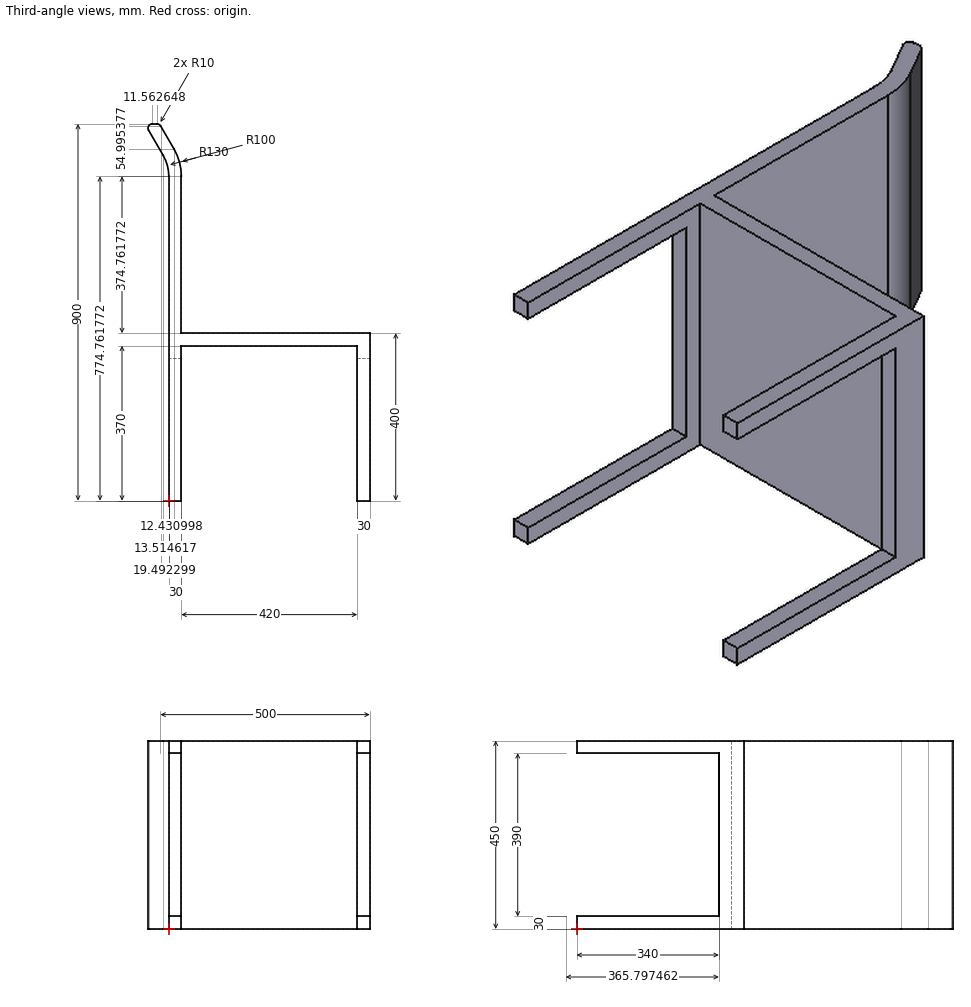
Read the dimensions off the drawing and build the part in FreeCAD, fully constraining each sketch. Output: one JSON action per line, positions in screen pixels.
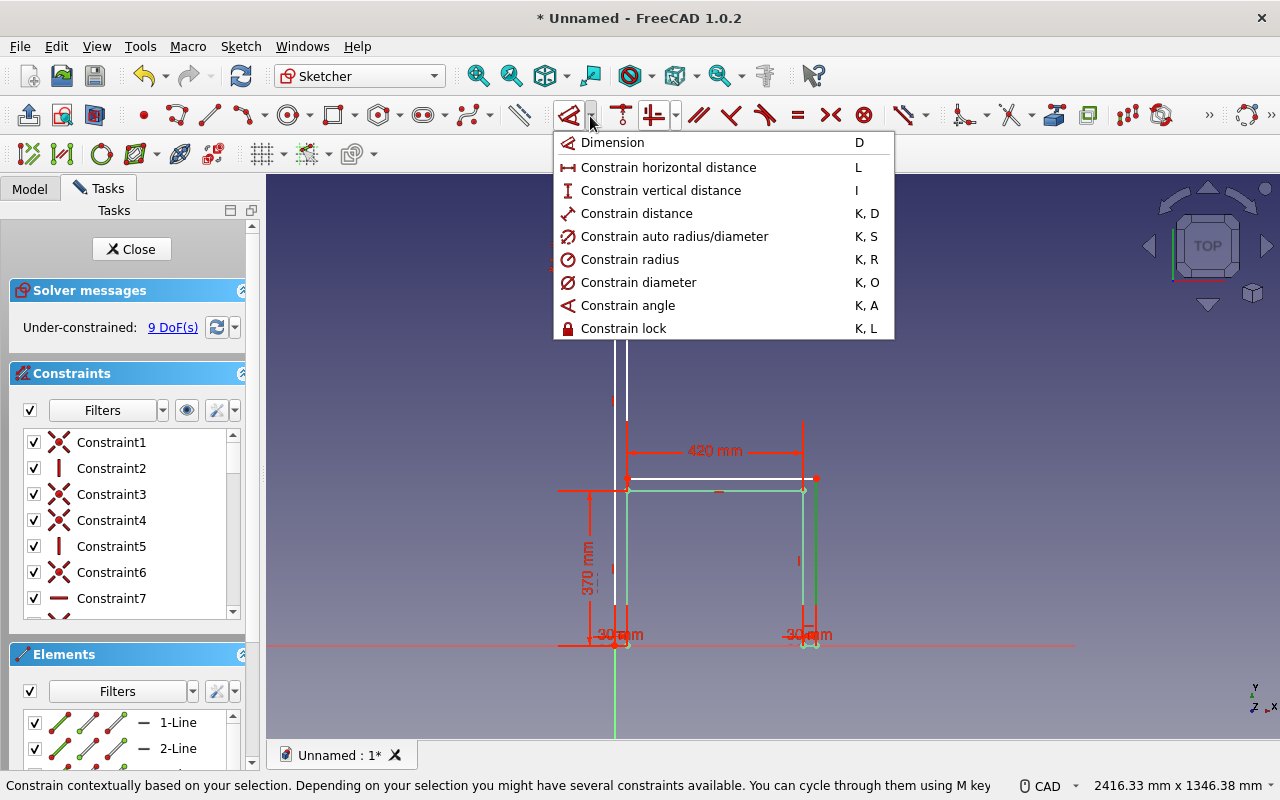
{"action": "left_click", "coordinate": [724, 190]}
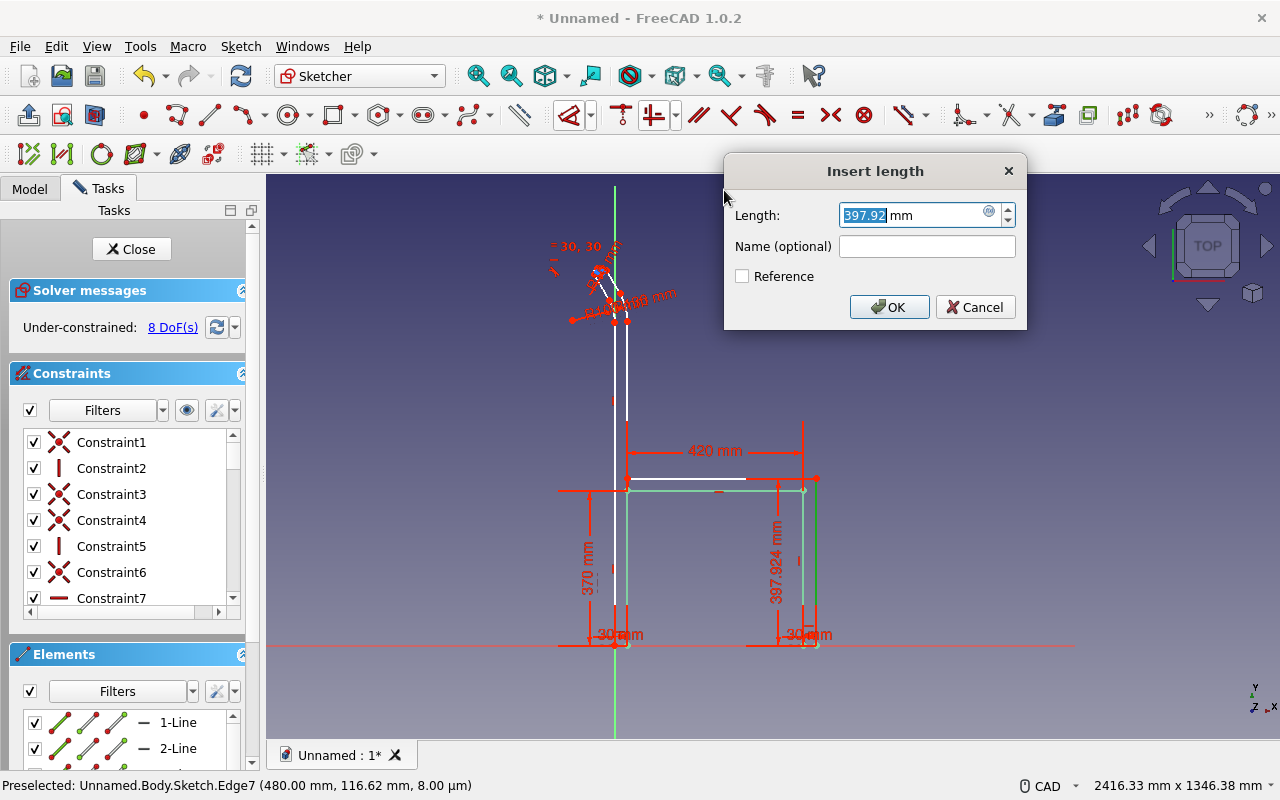
{"action": "type", "text": "400"}
{"action": "key", "text": "Return"}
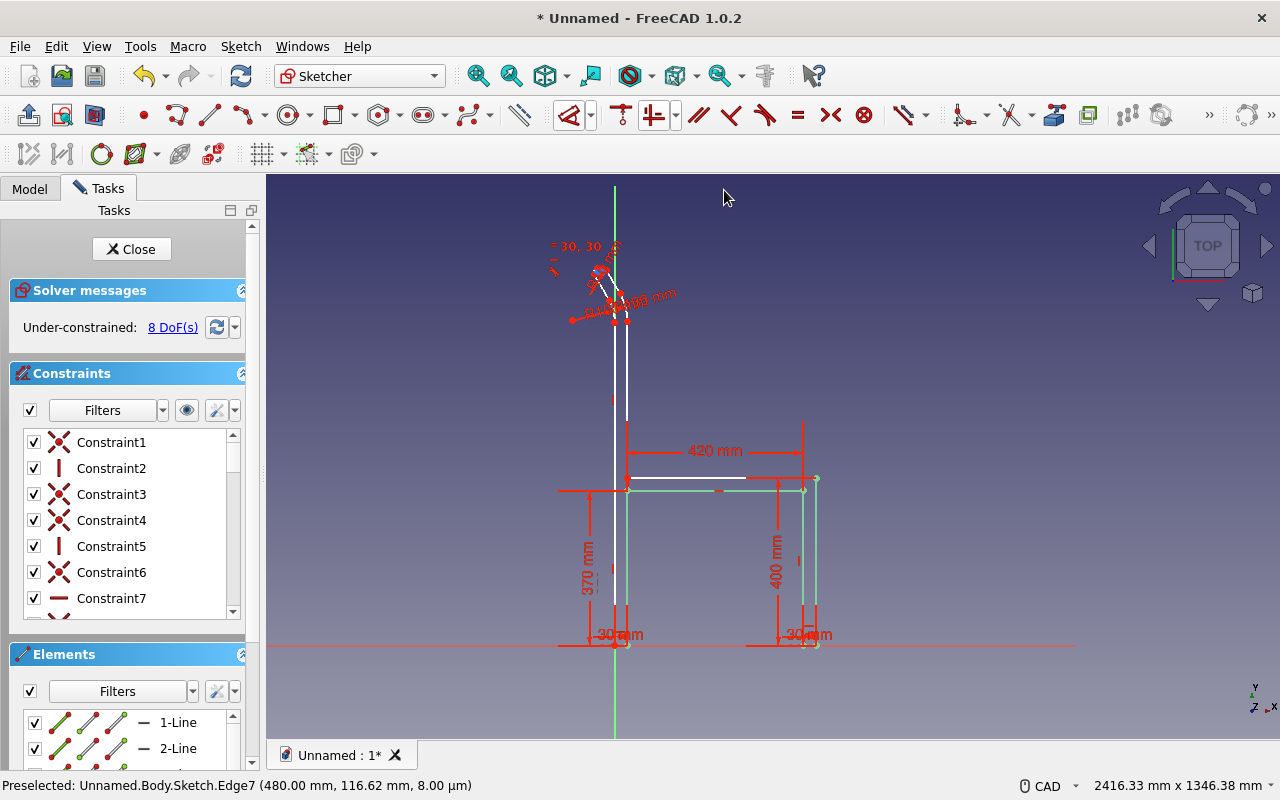
{"action": "scroll", "coordinate": [603, 269], "scroll_direction": "up", "scroll_amount": 6}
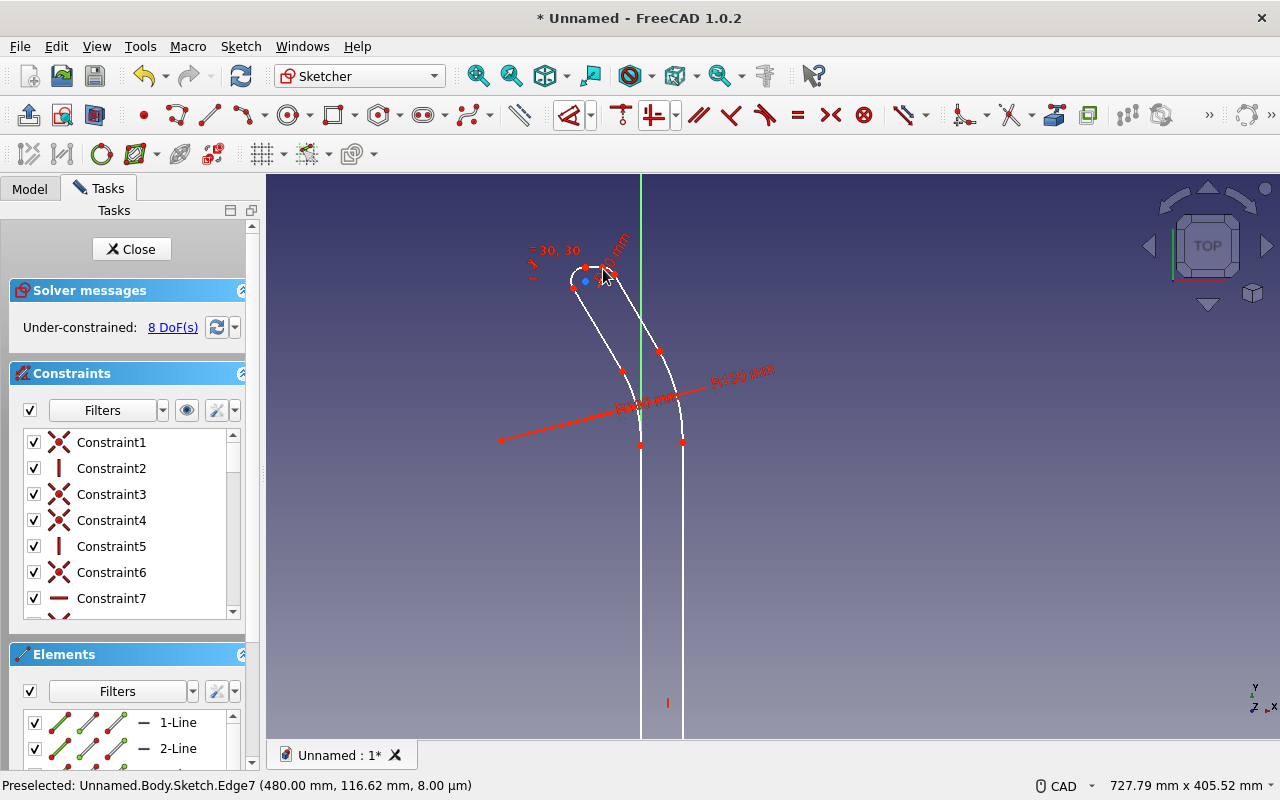
{"action": "left_click", "coordinate": [602, 267]}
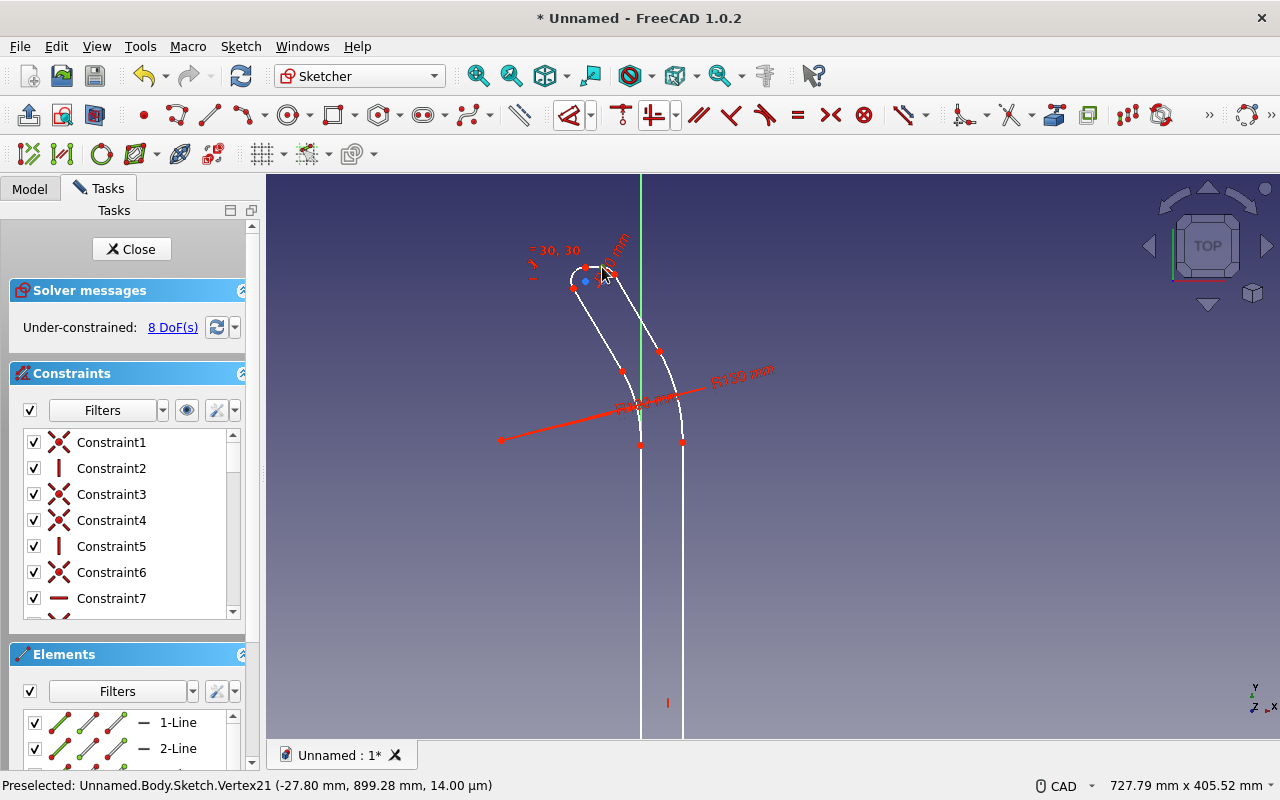
{"action": "key", "text": "i"}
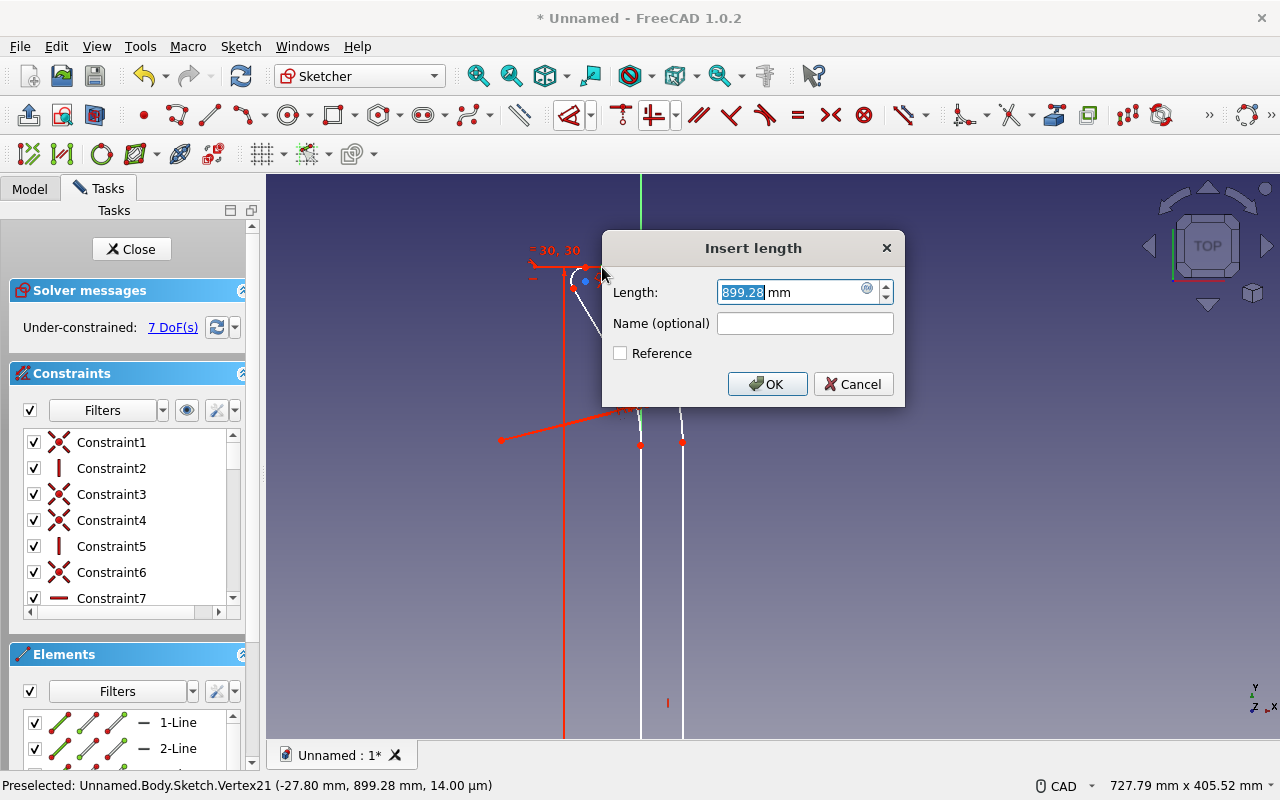
{"action": "type", "text": "900"}
{"action": "key", "text": "Return"}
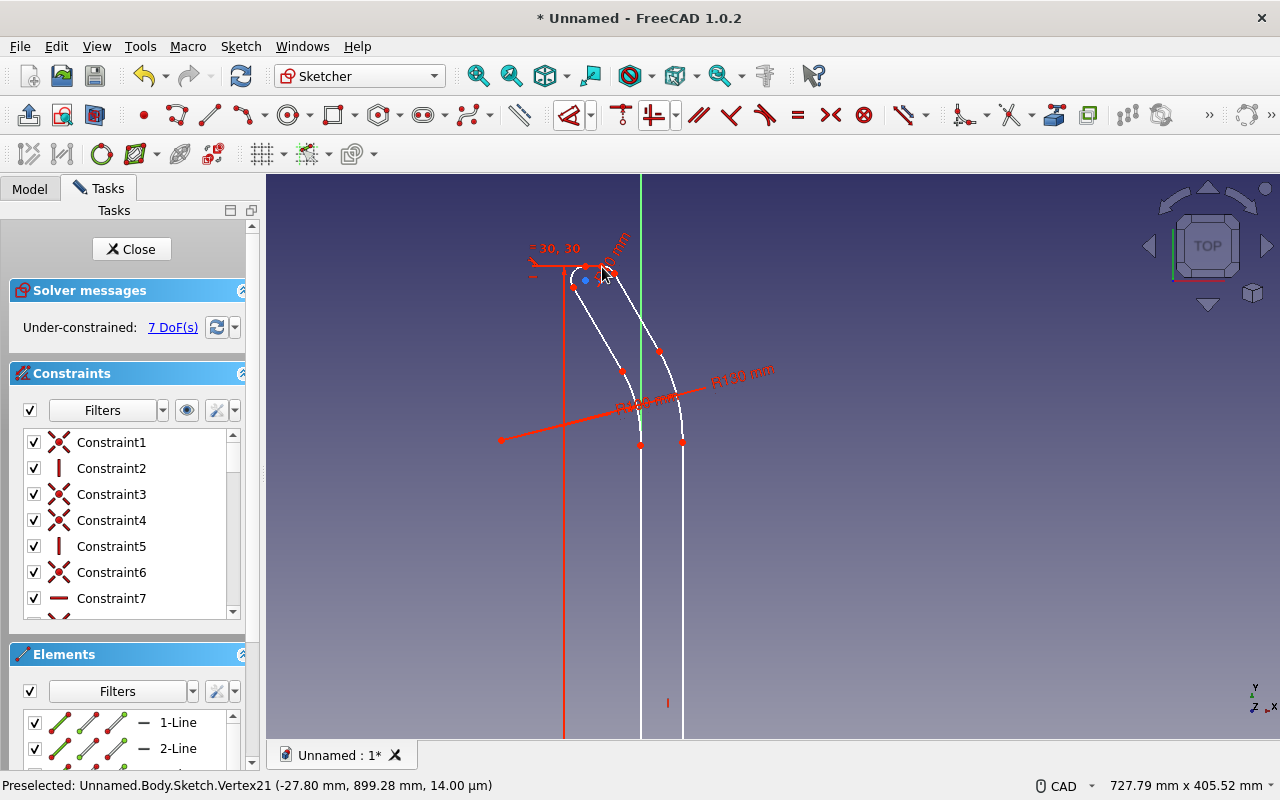
{"action": "scroll", "coordinate": [594, 266], "scroll_direction": "up", "scroll_amount": 5}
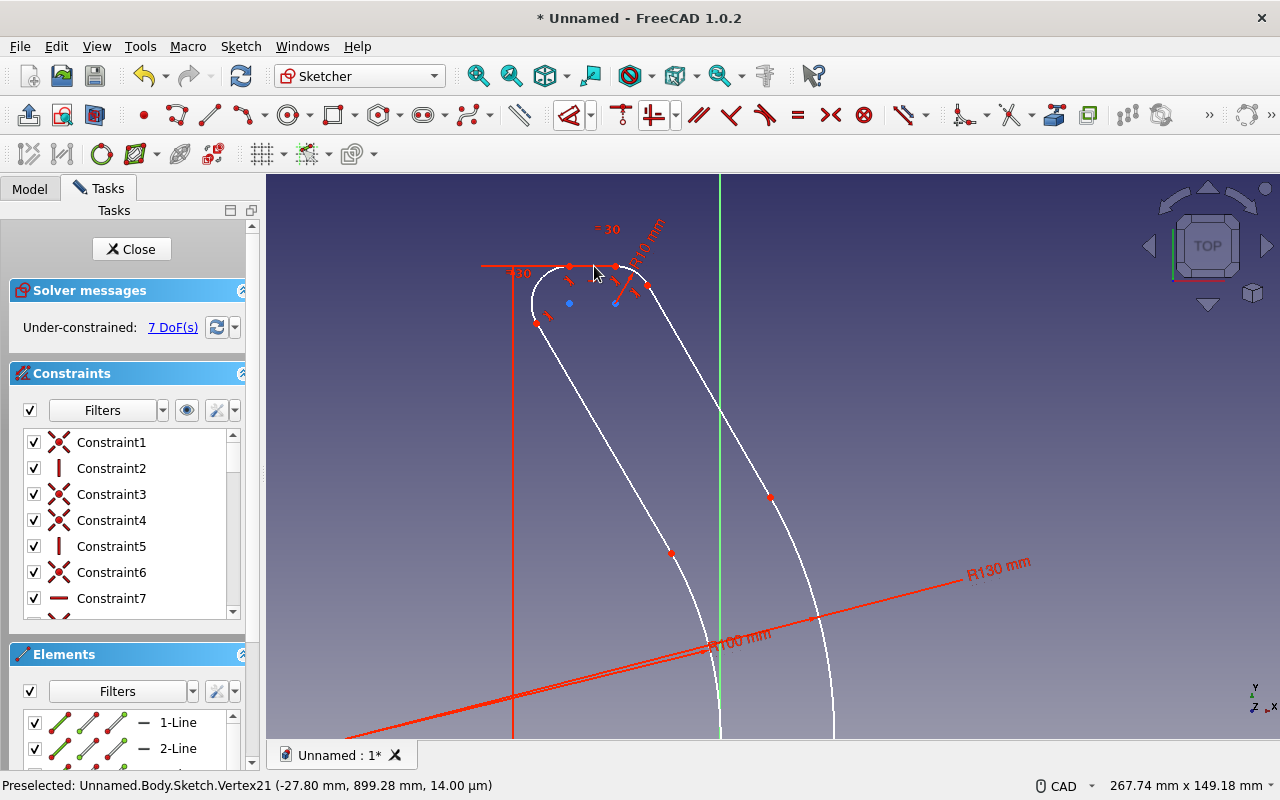
{"action": "left_click", "coordinate": [592, 266]}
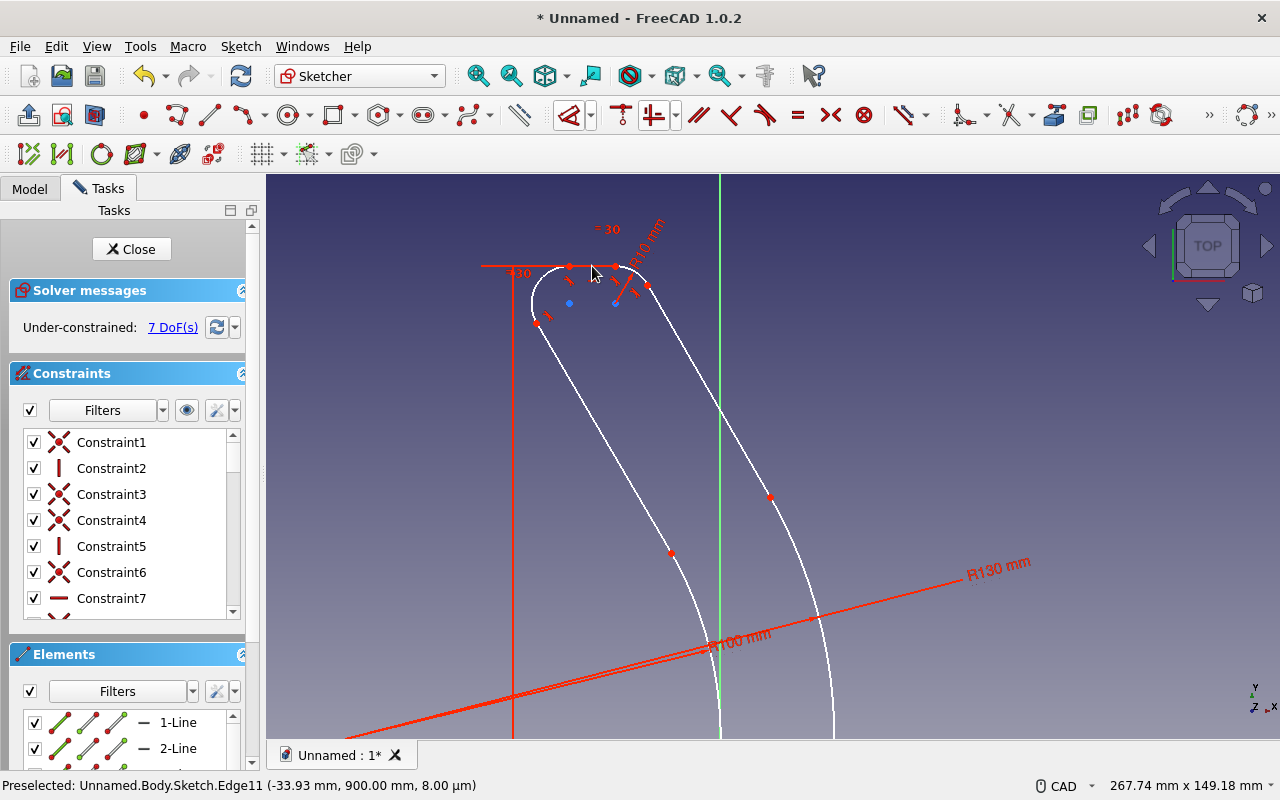
{"action": "key", "text": "l"}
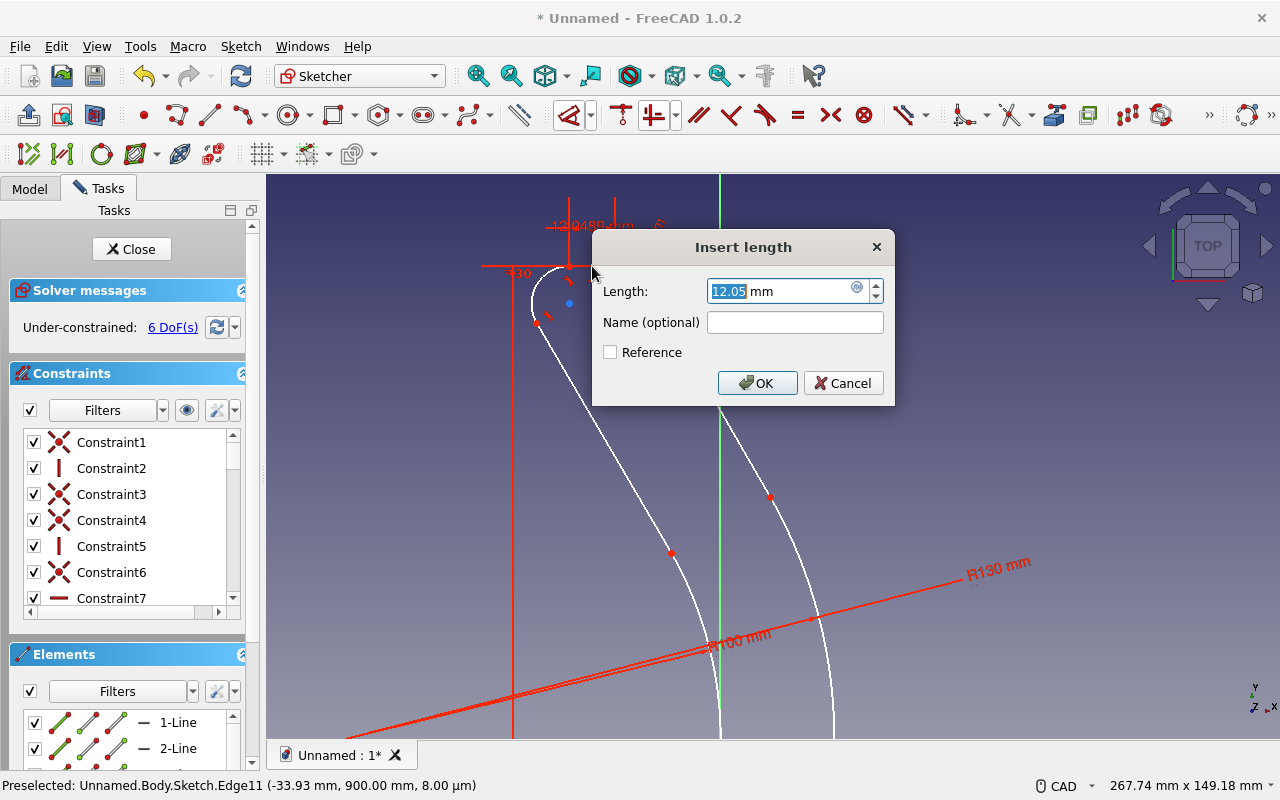
{"action": "type", "text": "11.562648"}
{"action": "key", "text": "Return"}